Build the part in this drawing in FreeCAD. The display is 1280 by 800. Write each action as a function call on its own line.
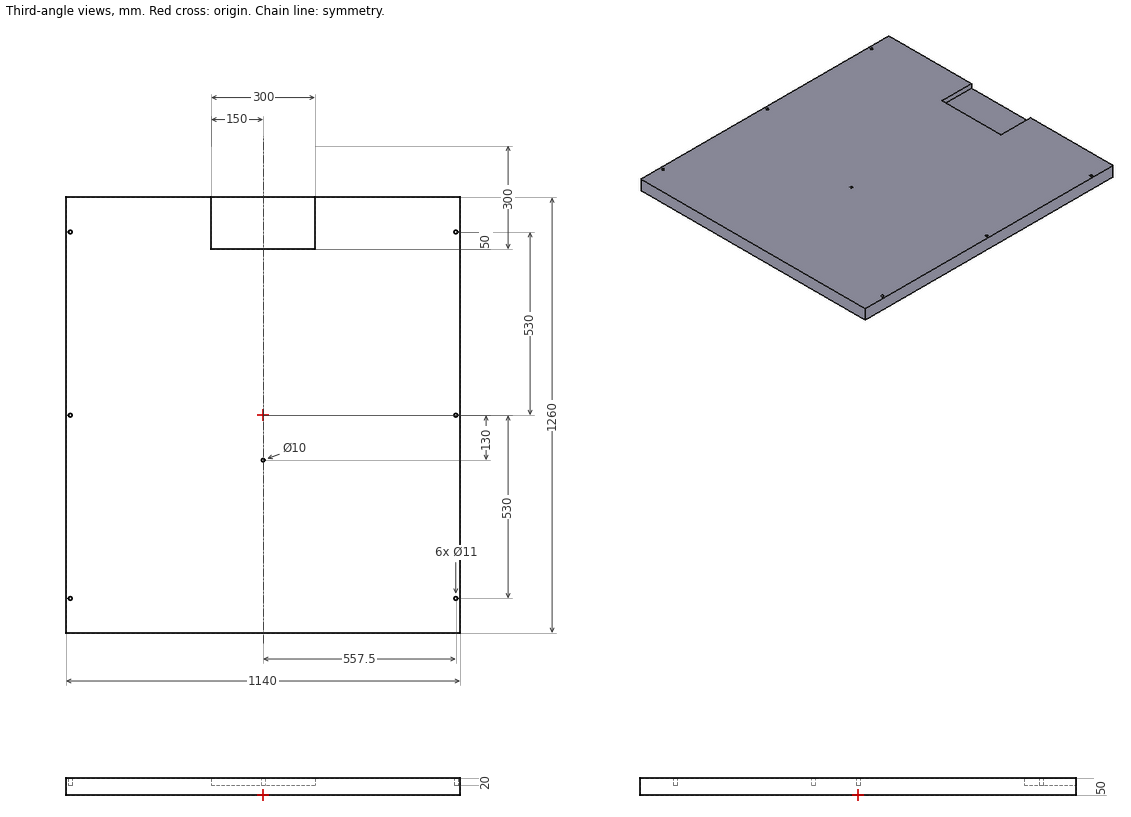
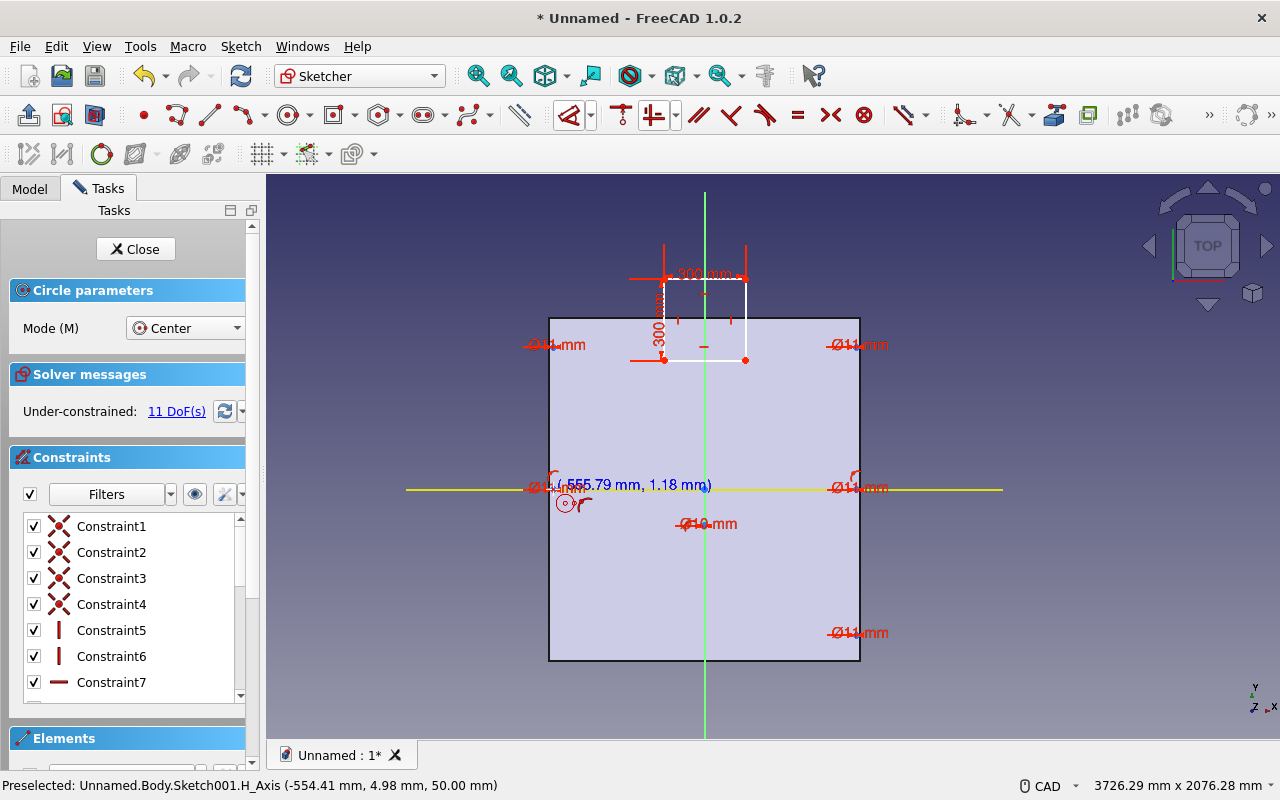
scroll(553, 634, up, 14)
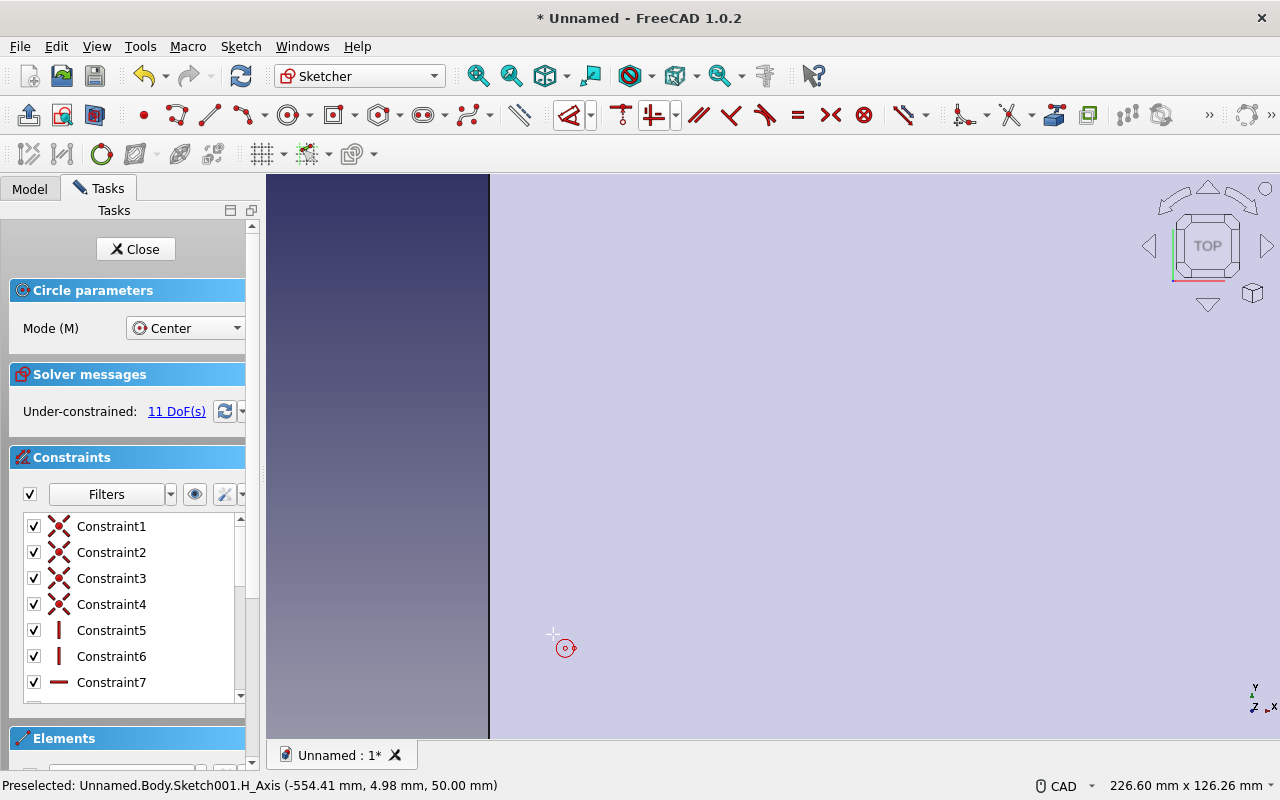
scroll(553, 635, down, 14)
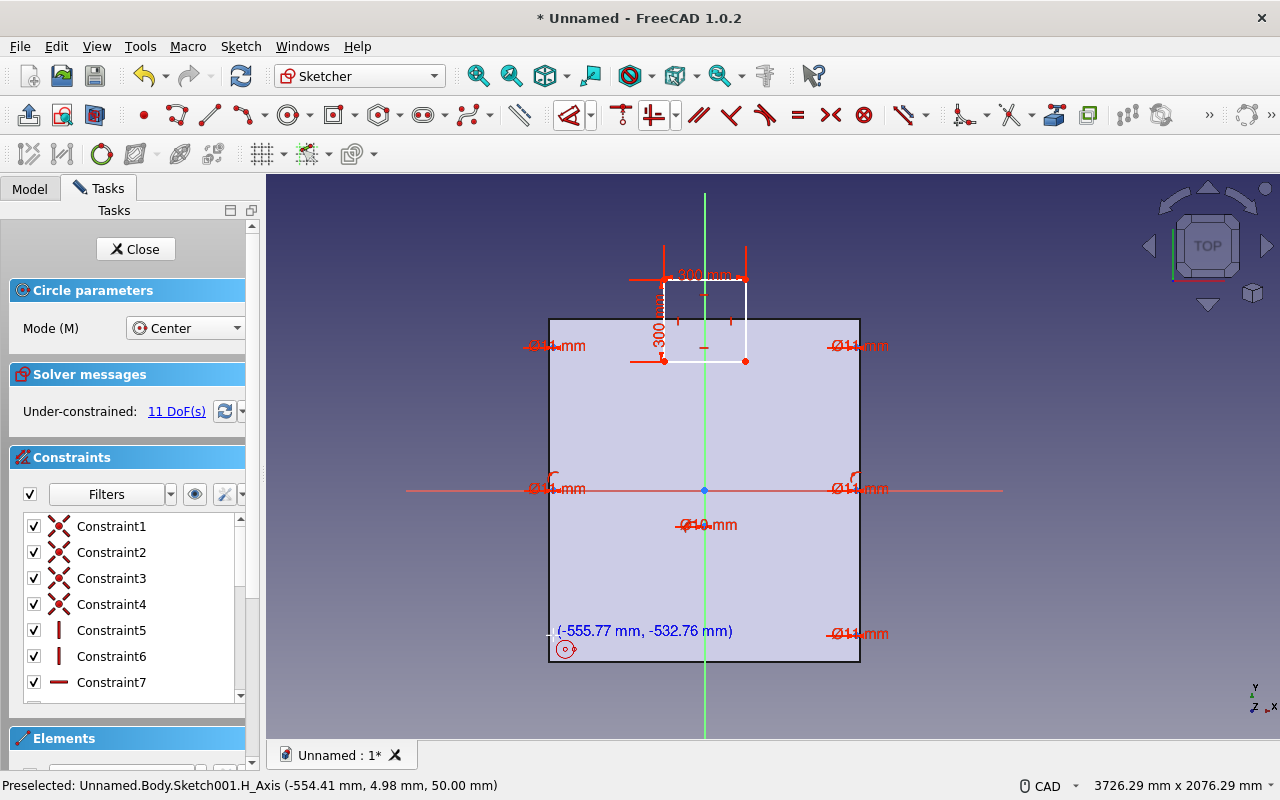
click(553, 635)
move(554, 634)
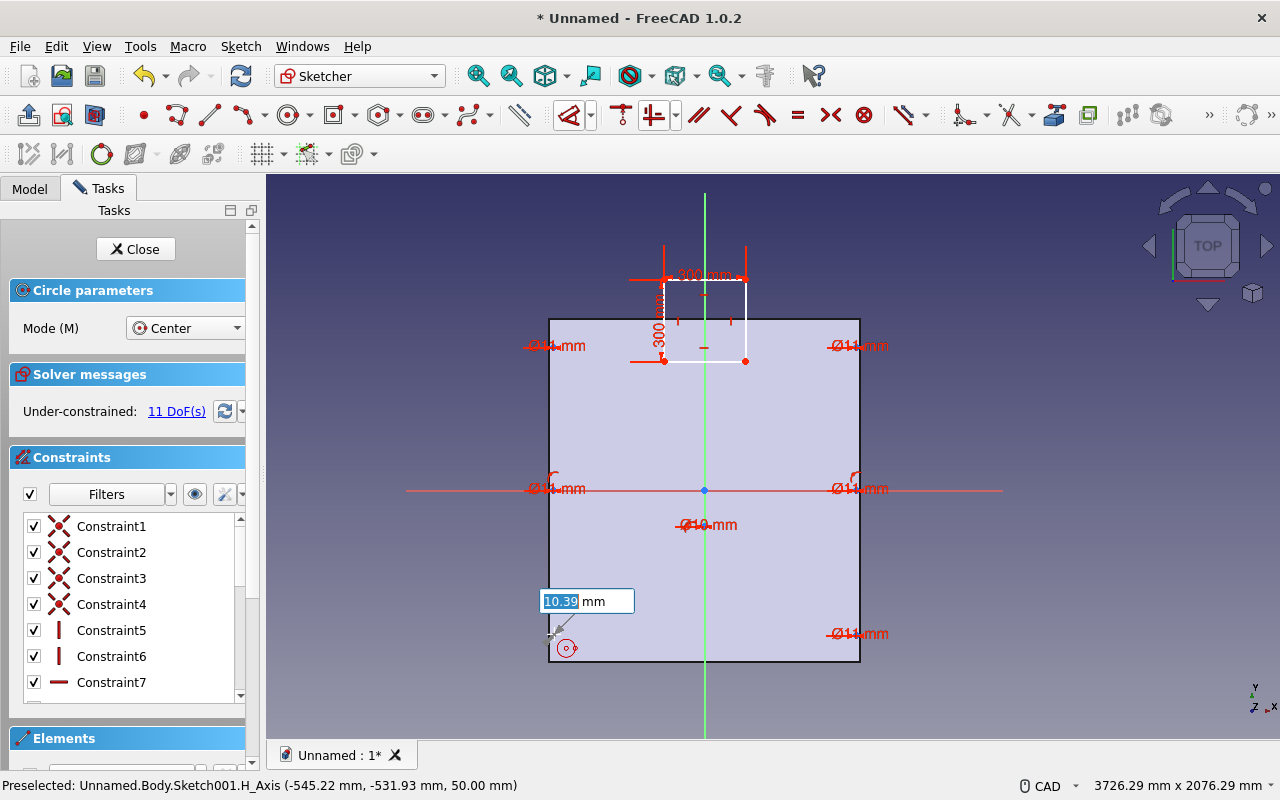
text(11)
key(Return)
key(Escape)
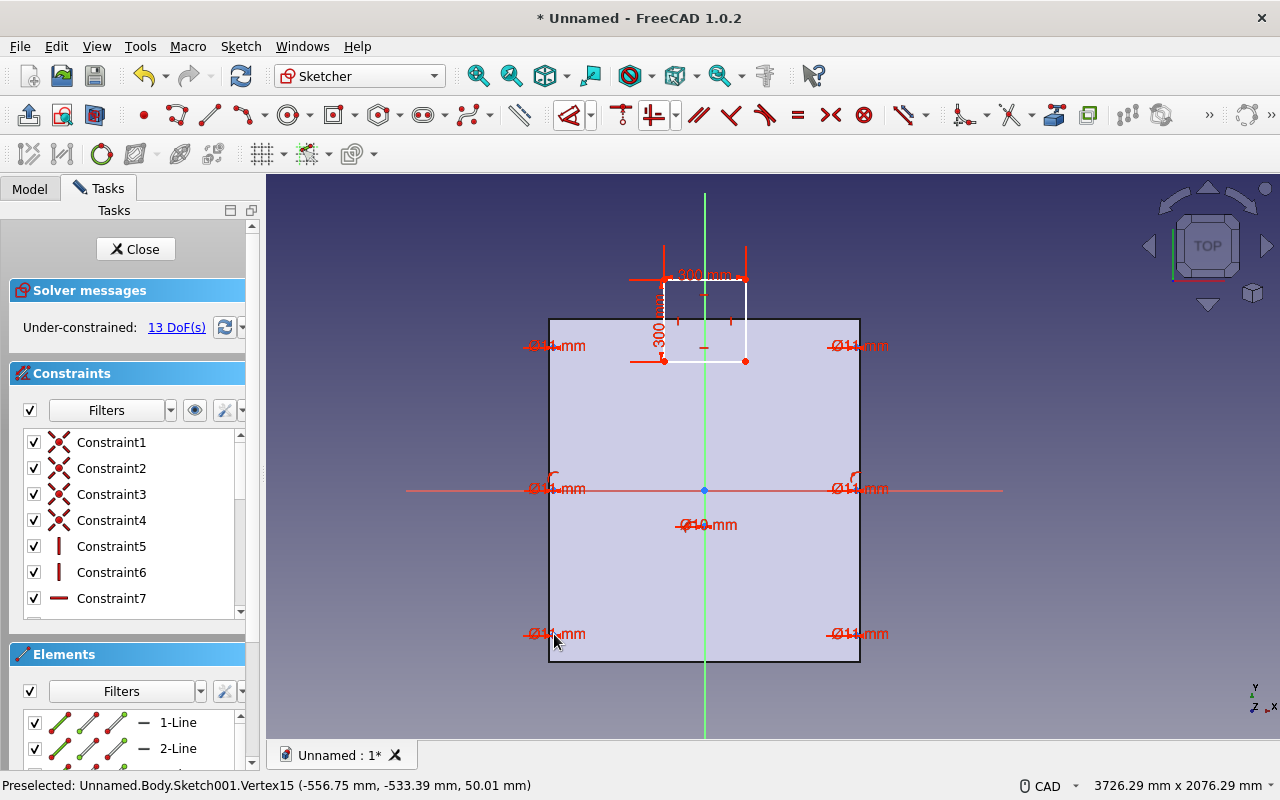
click(856, 636)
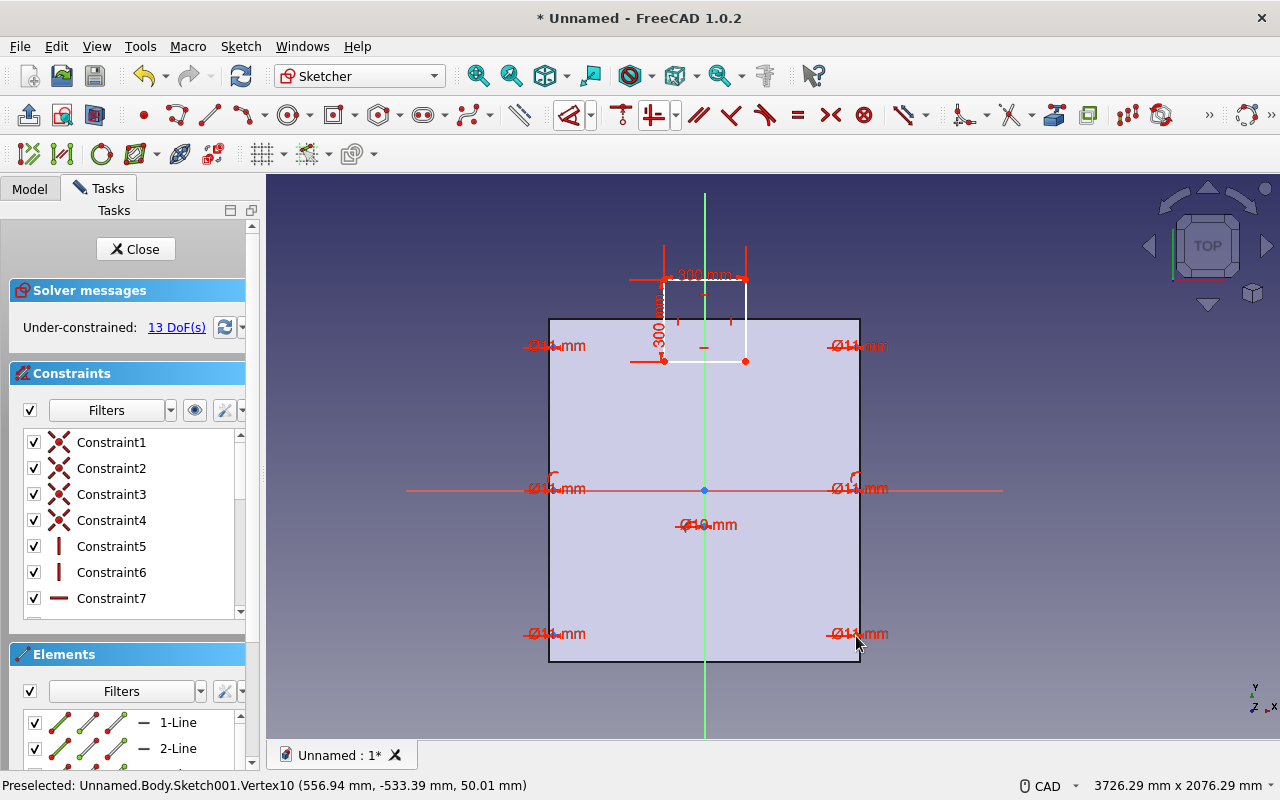
click(856, 491)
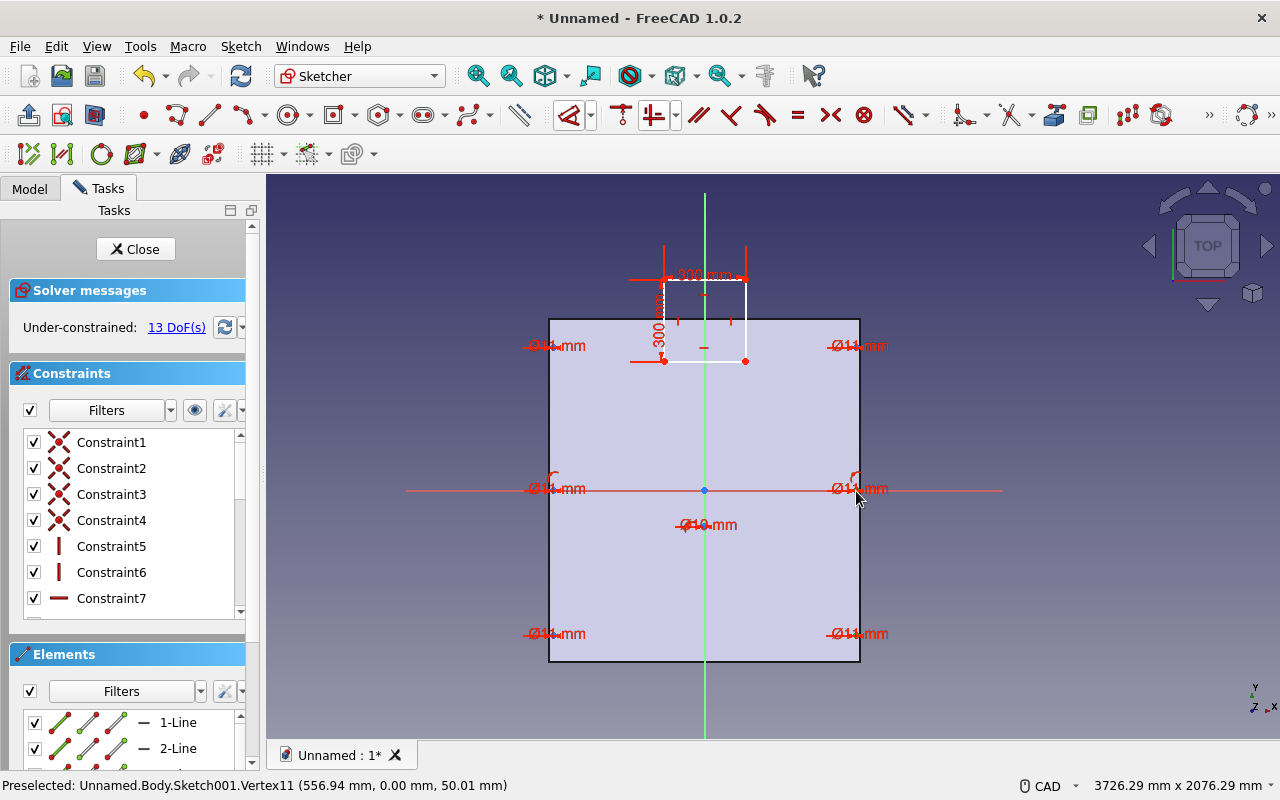
click(676, 116)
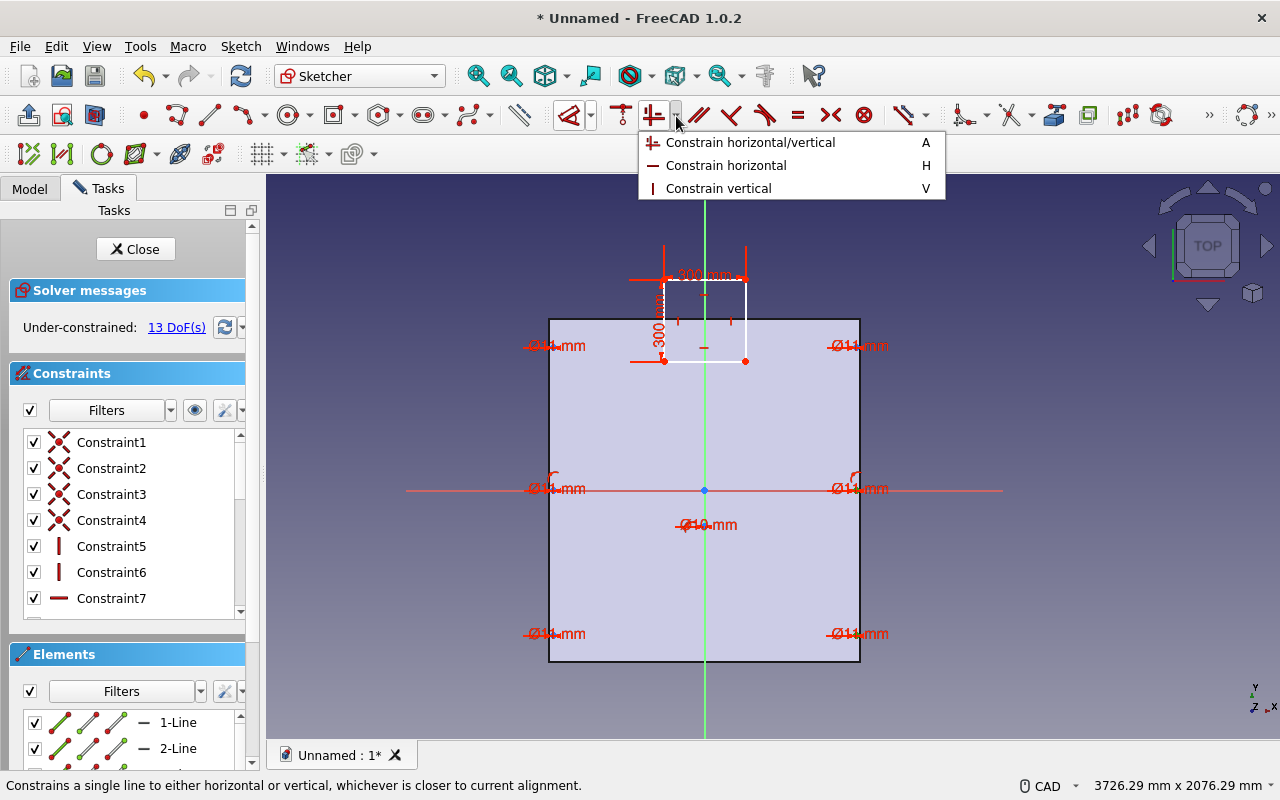
click(792, 188)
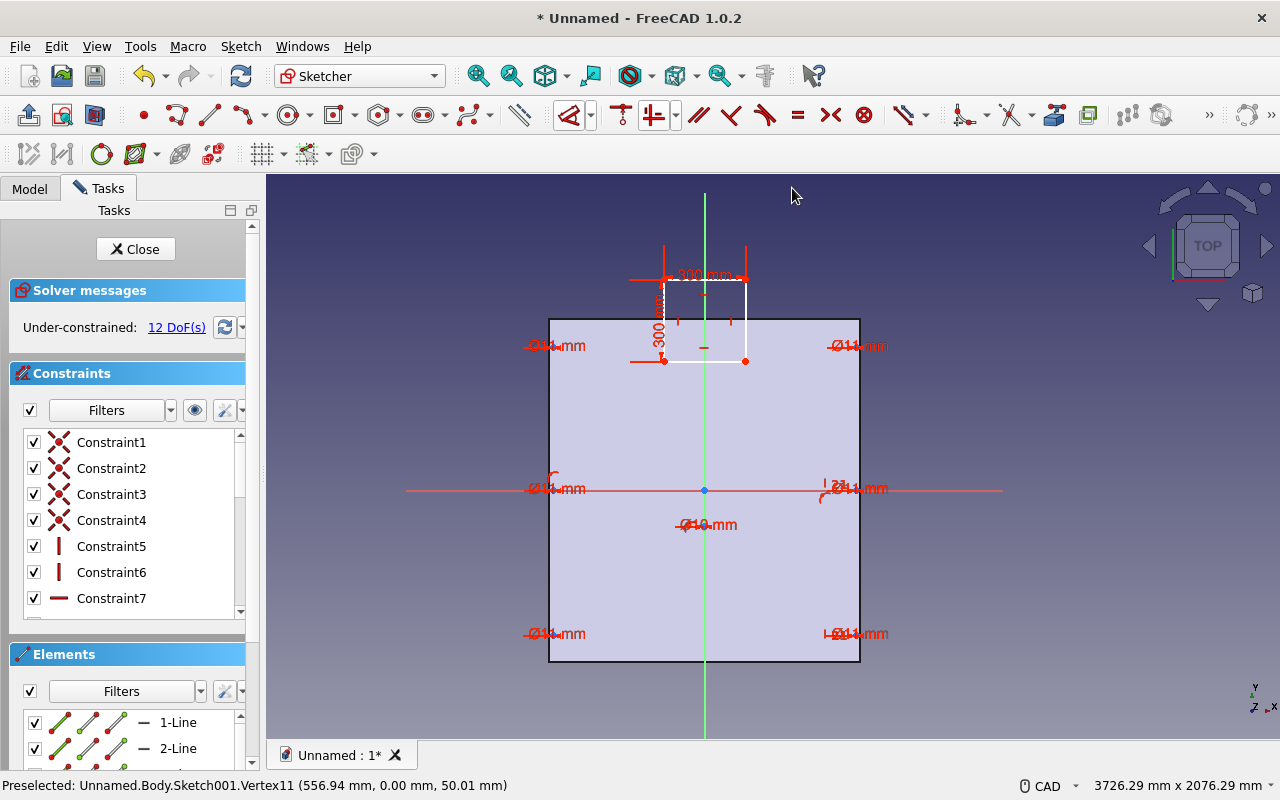
click(856, 491)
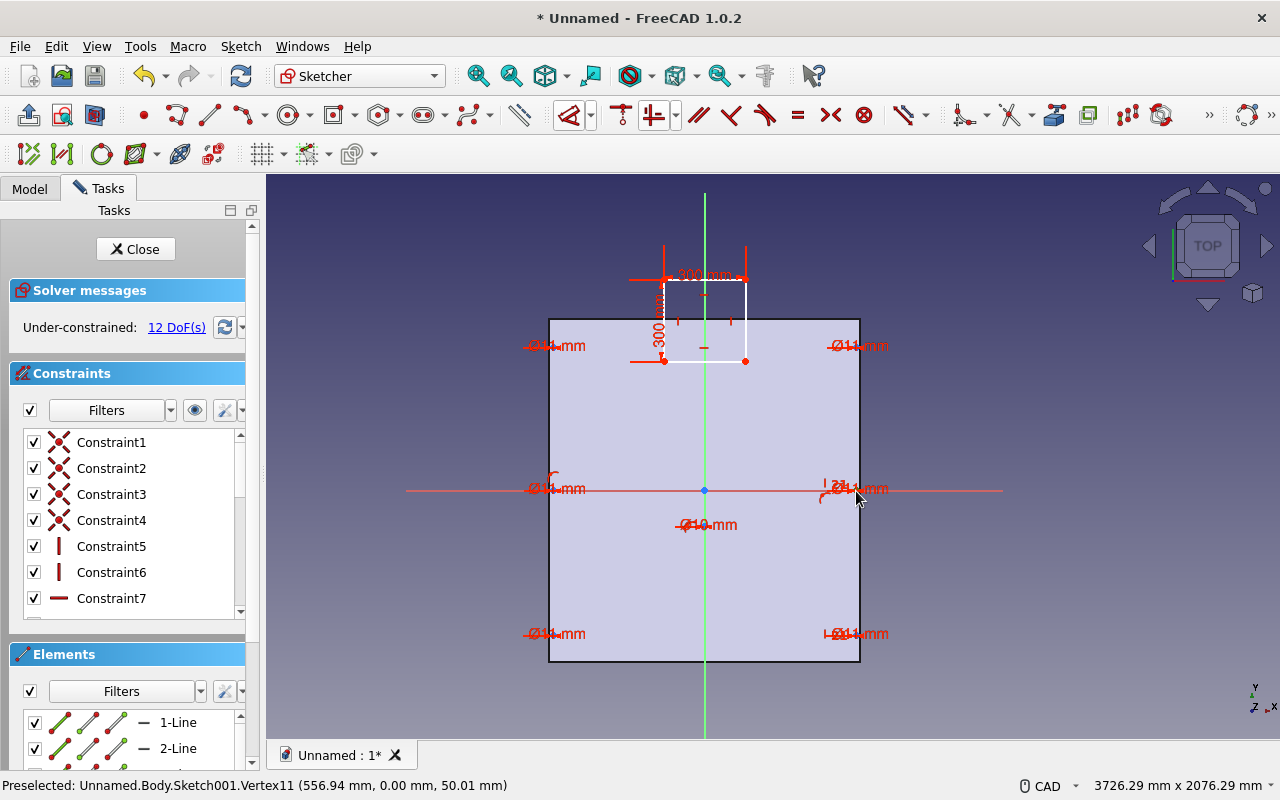
click(856, 348)